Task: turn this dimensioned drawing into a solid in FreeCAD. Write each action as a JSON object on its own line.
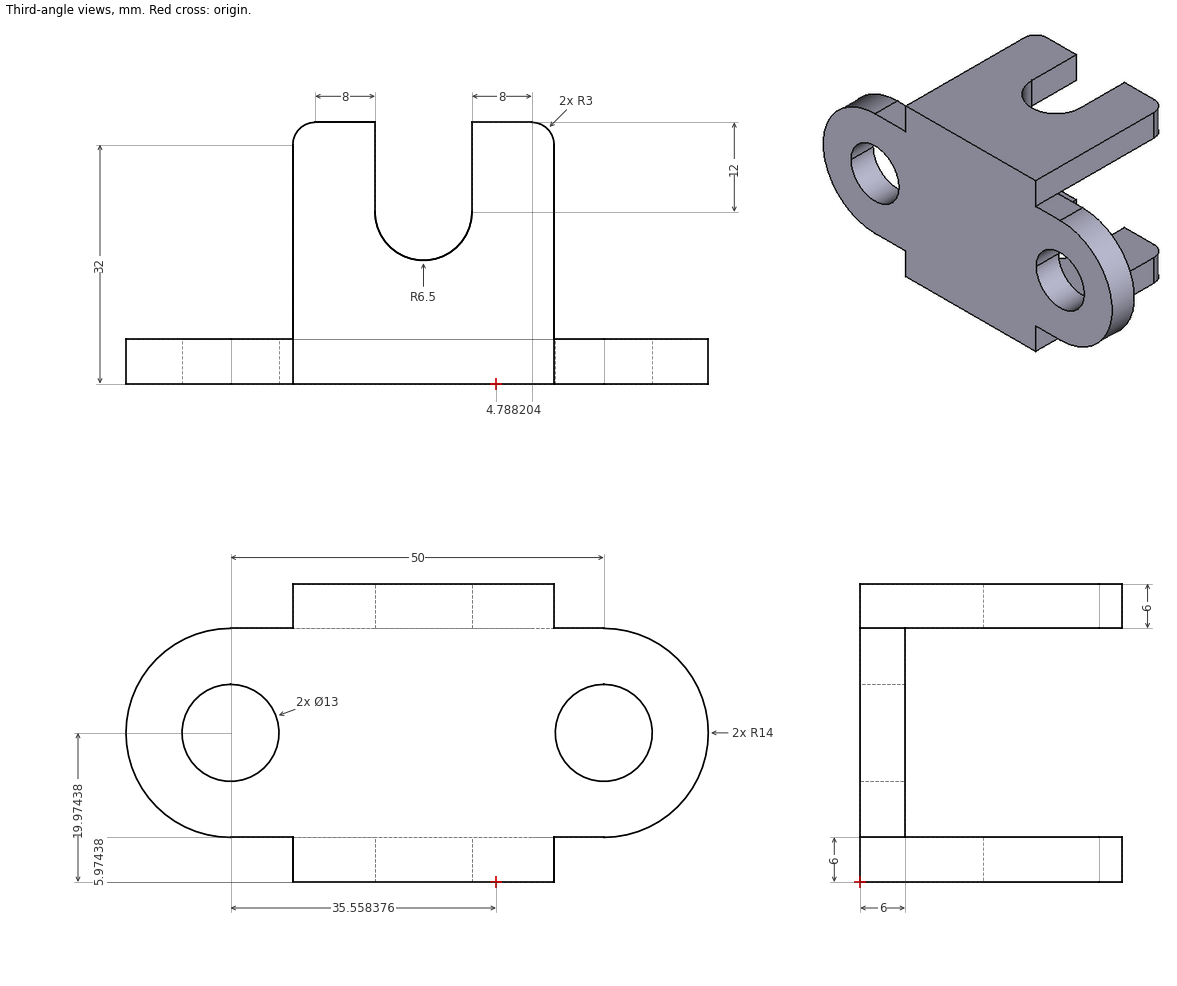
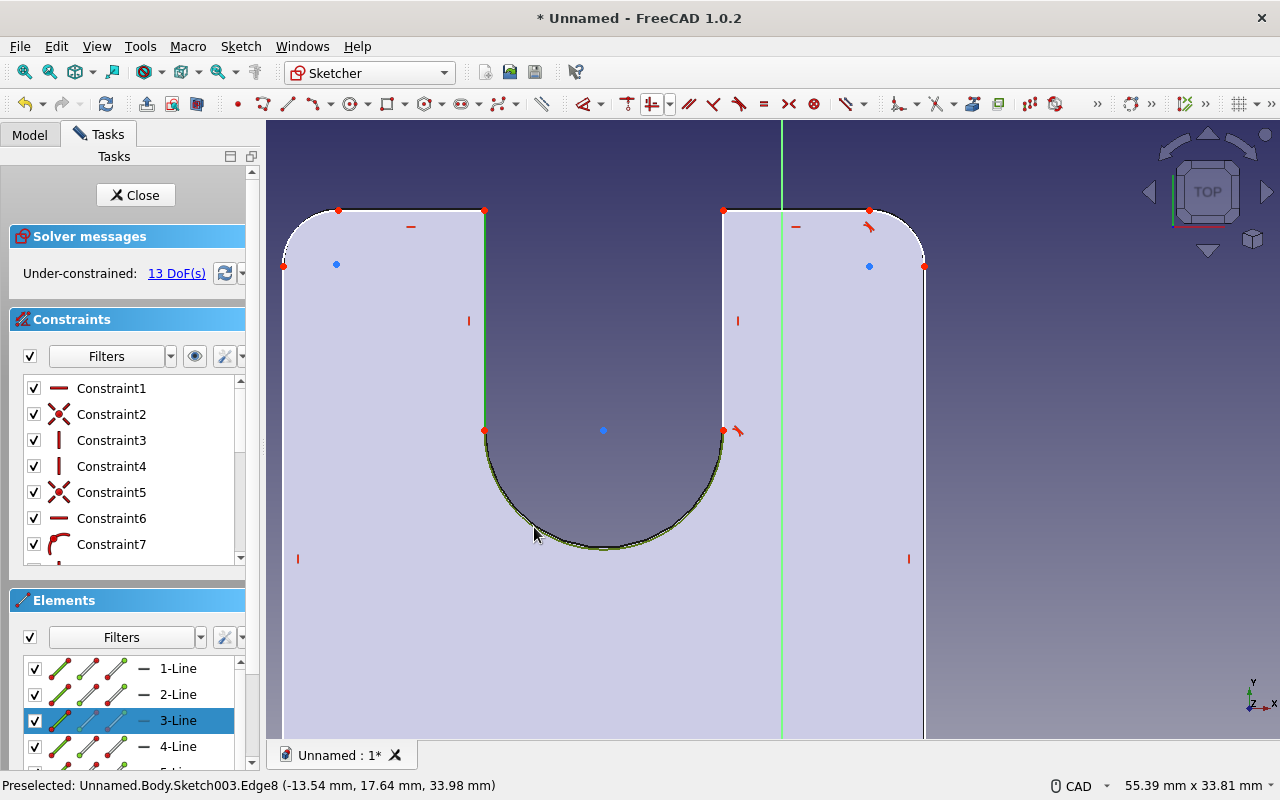
{"action": "left_click", "coordinate": [739, 104]}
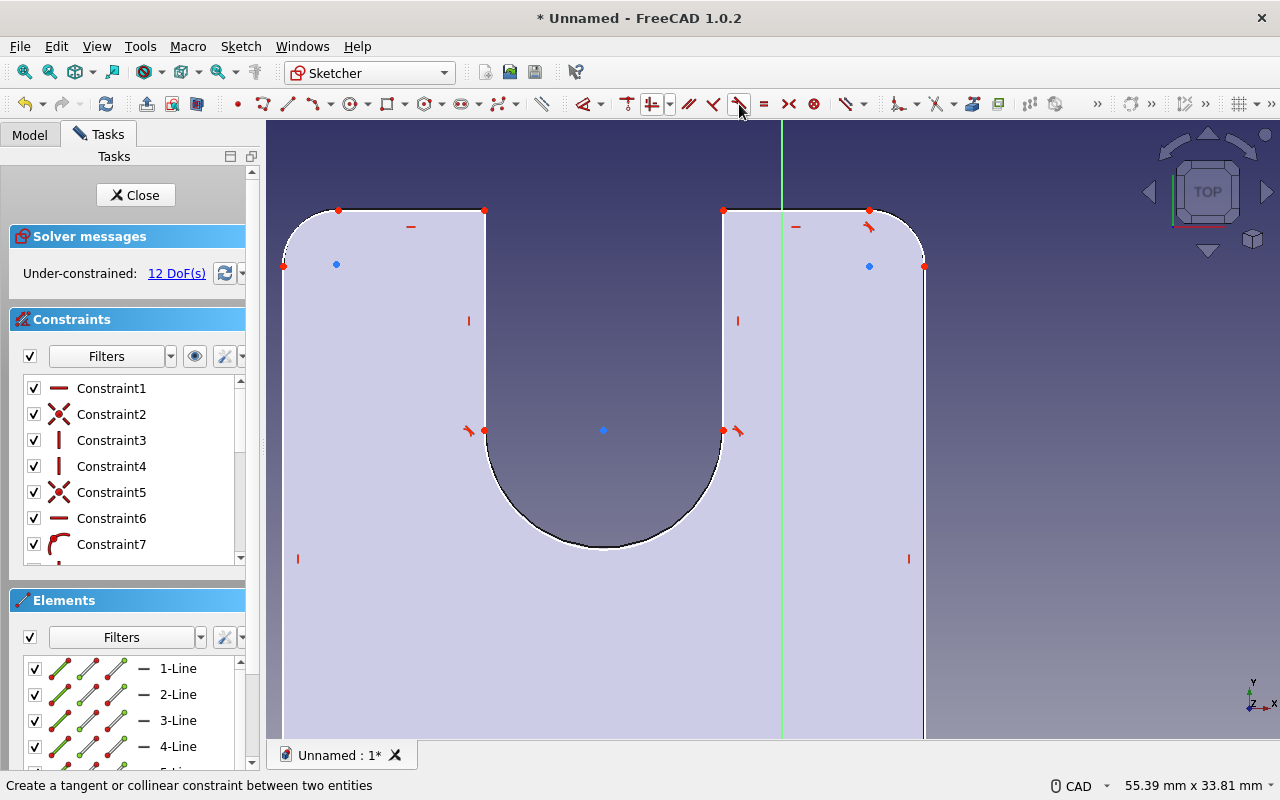
{"action": "left_click", "coordinate": [441, 211]}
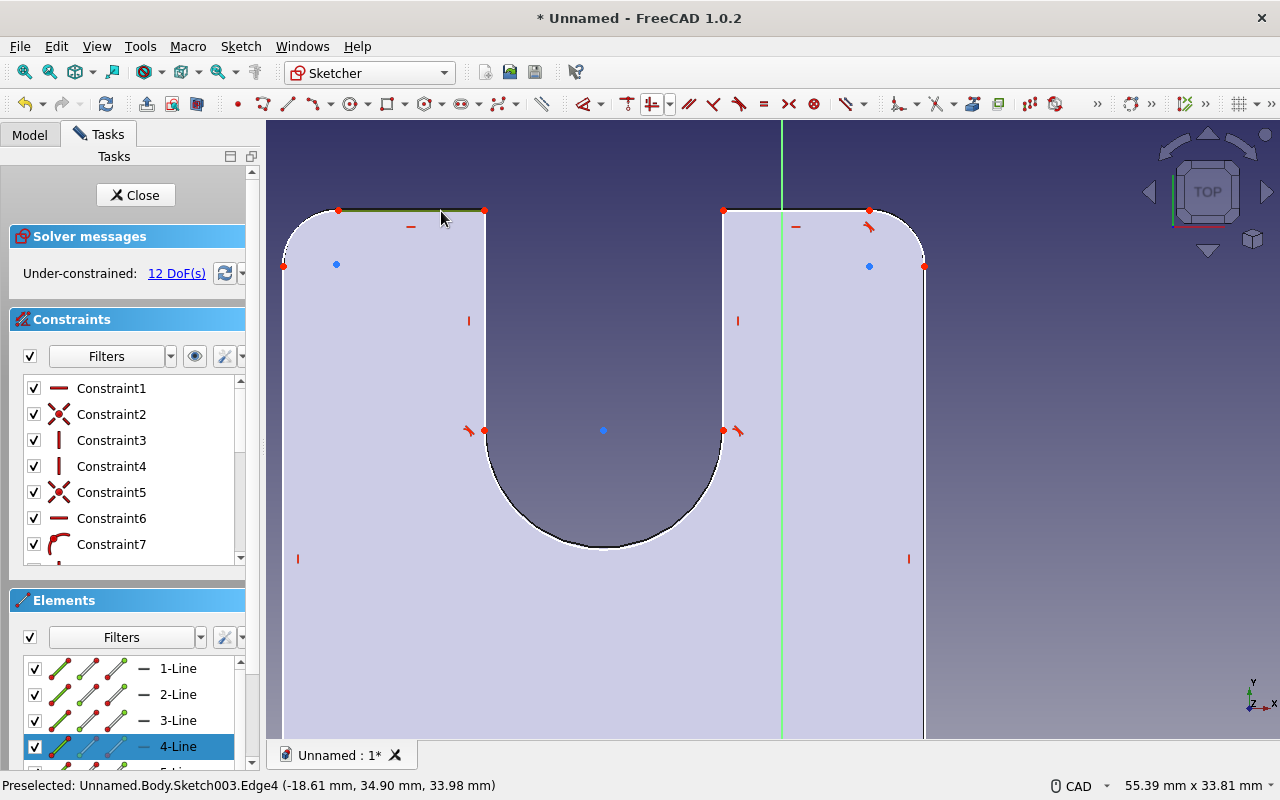
{"action": "left_click", "coordinate": [313, 217]}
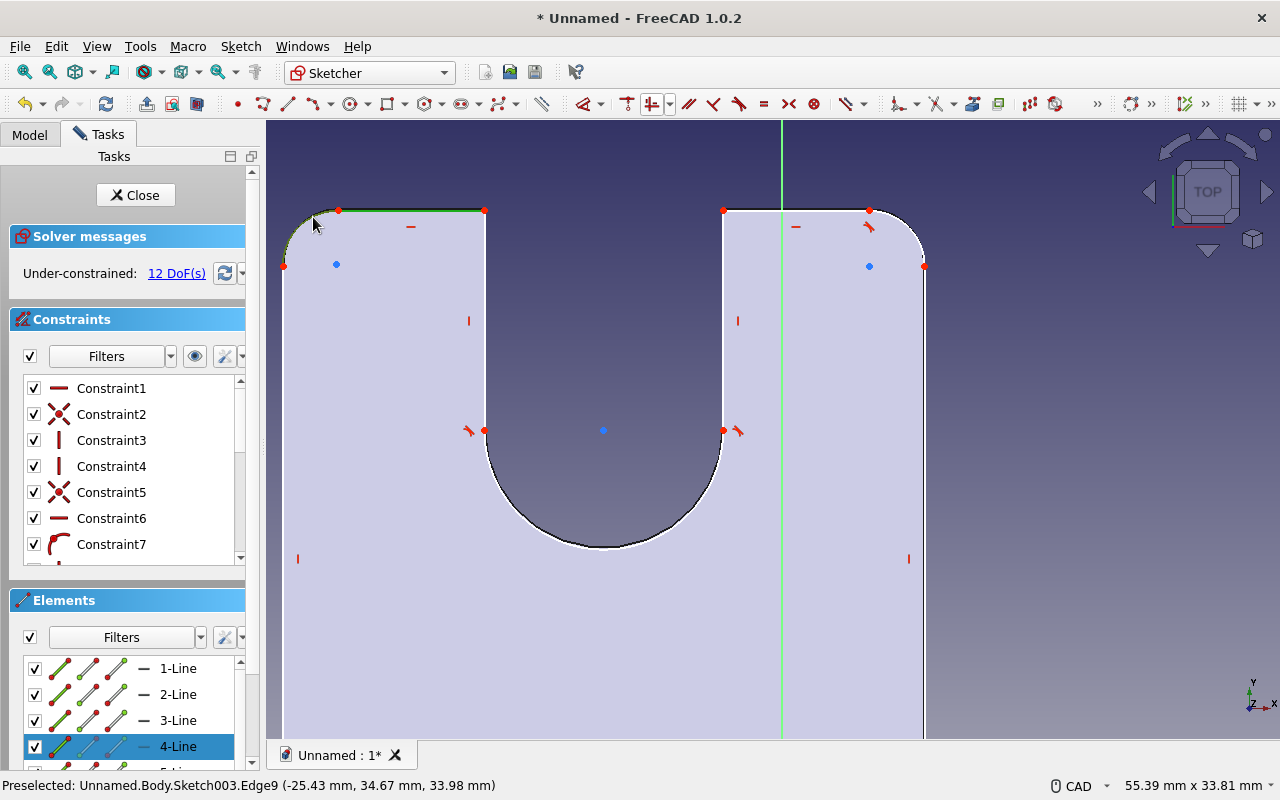
{"action": "left_click", "coordinate": [739, 104]}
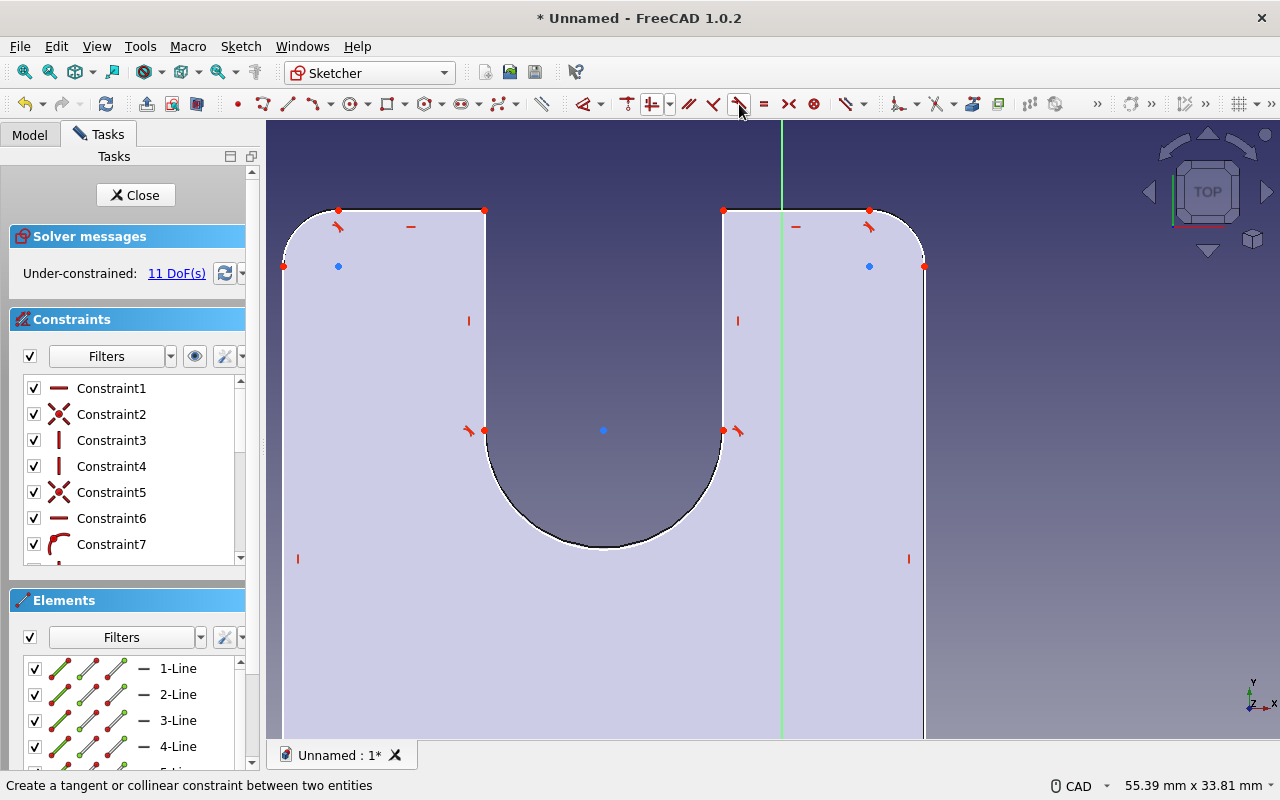
{"action": "scroll", "coordinate": [909, 226], "scroll_direction": "down", "scroll_amount": 2}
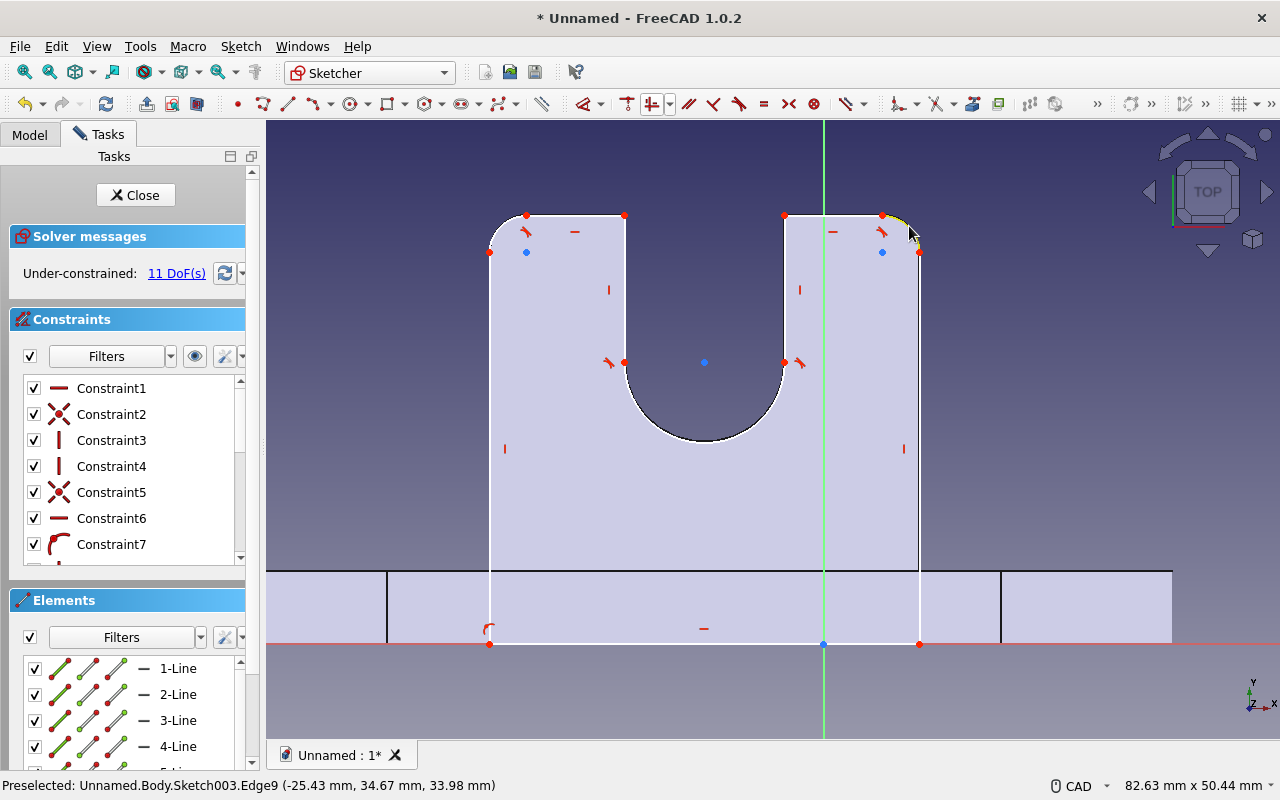
{"action": "left_click", "coordinate": [490, 370]}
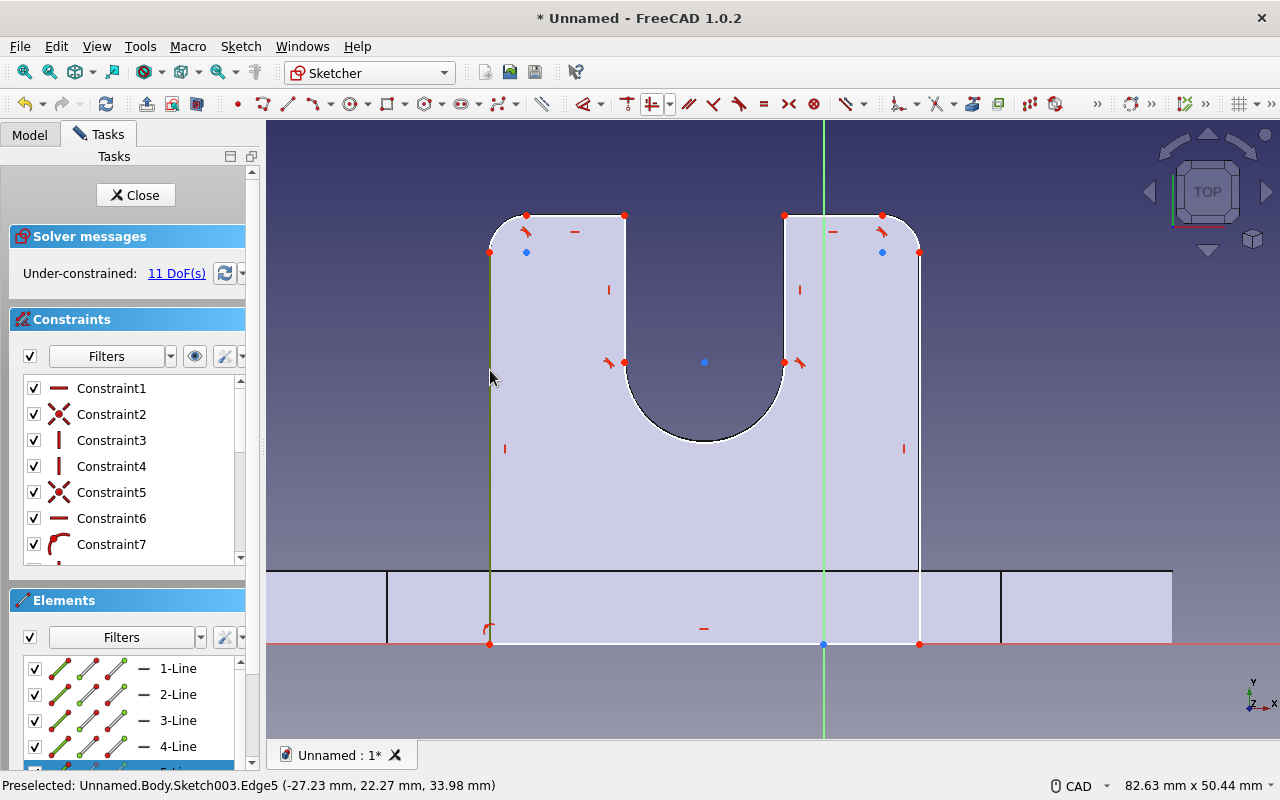
{"action": "left_click", "coordinate": [510, 220]}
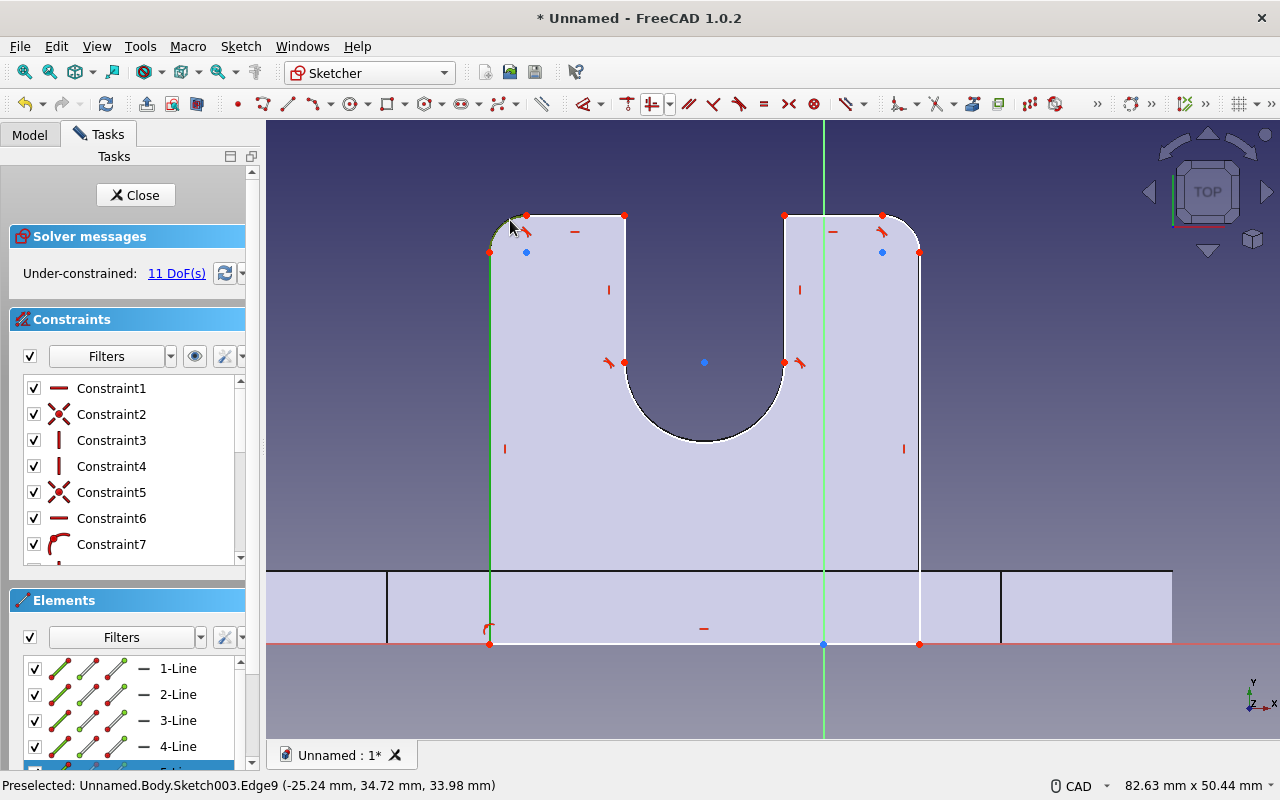
{"action": "left_click", "coordinate": [739, 104]}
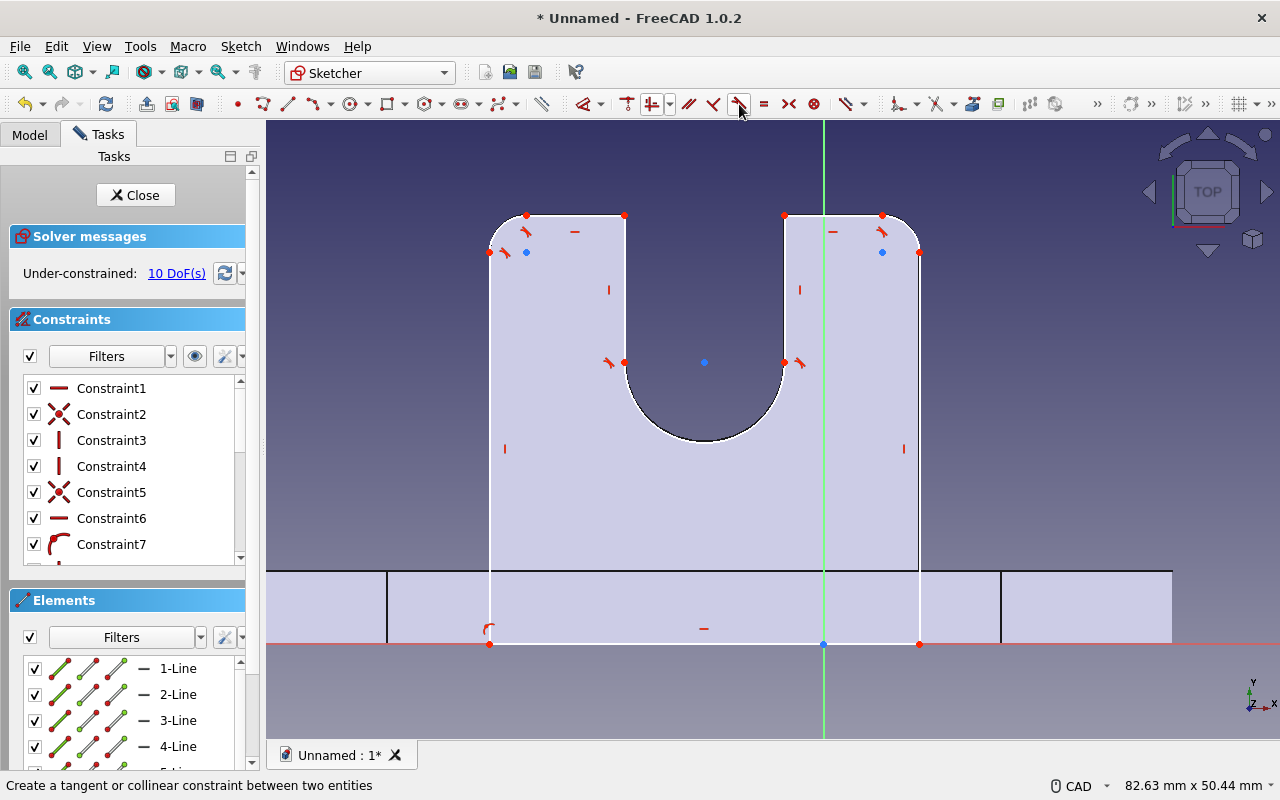
{"action": "left_click", "coordinate": [920, 527]}